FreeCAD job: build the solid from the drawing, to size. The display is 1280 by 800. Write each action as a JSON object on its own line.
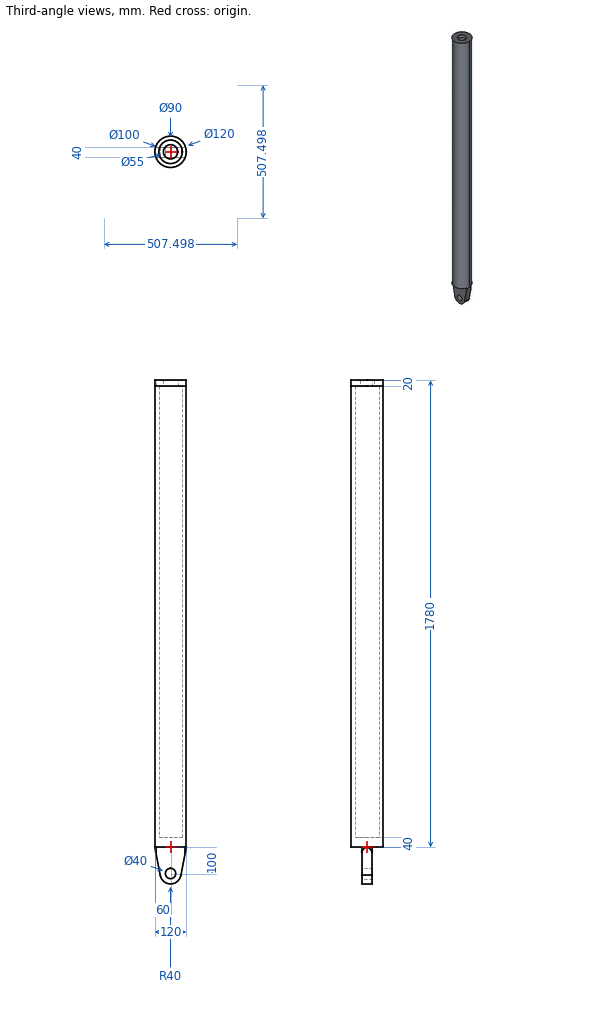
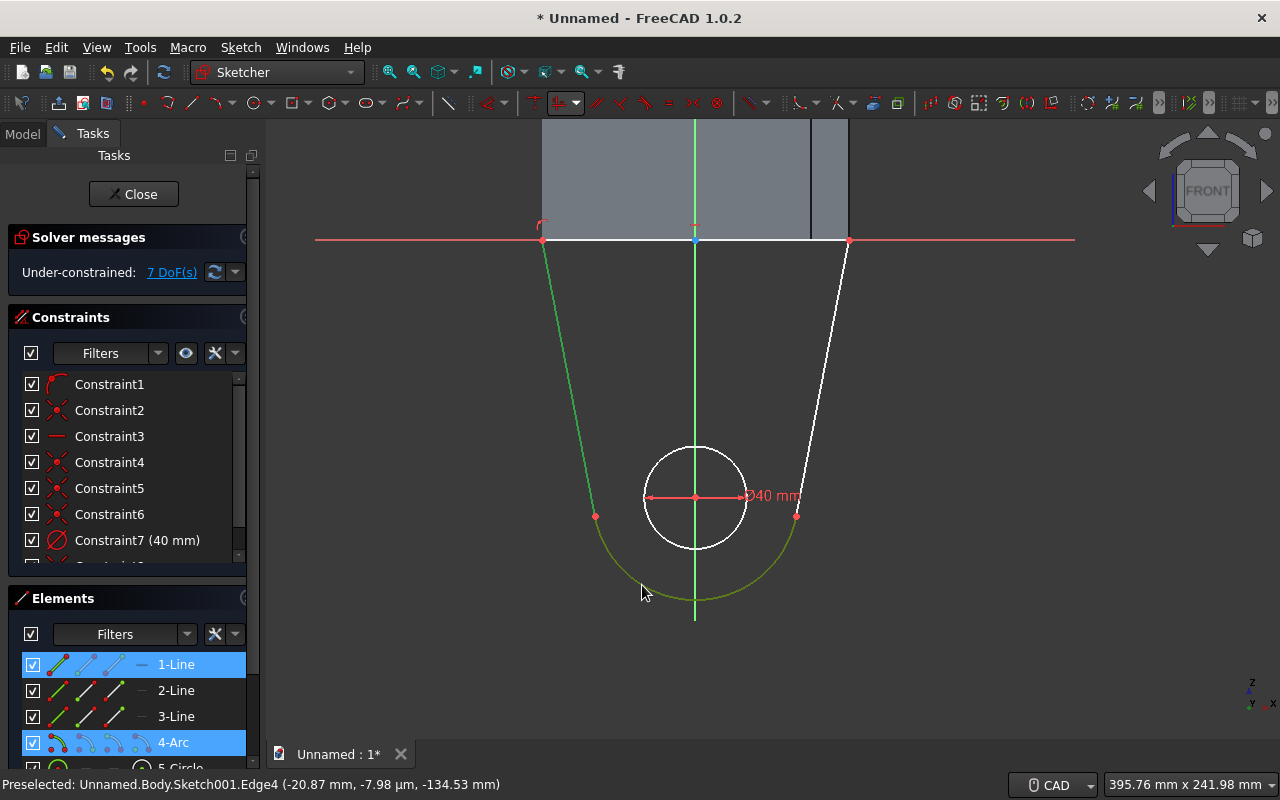
{"action": "left_click", "coordinate": [646, 104]}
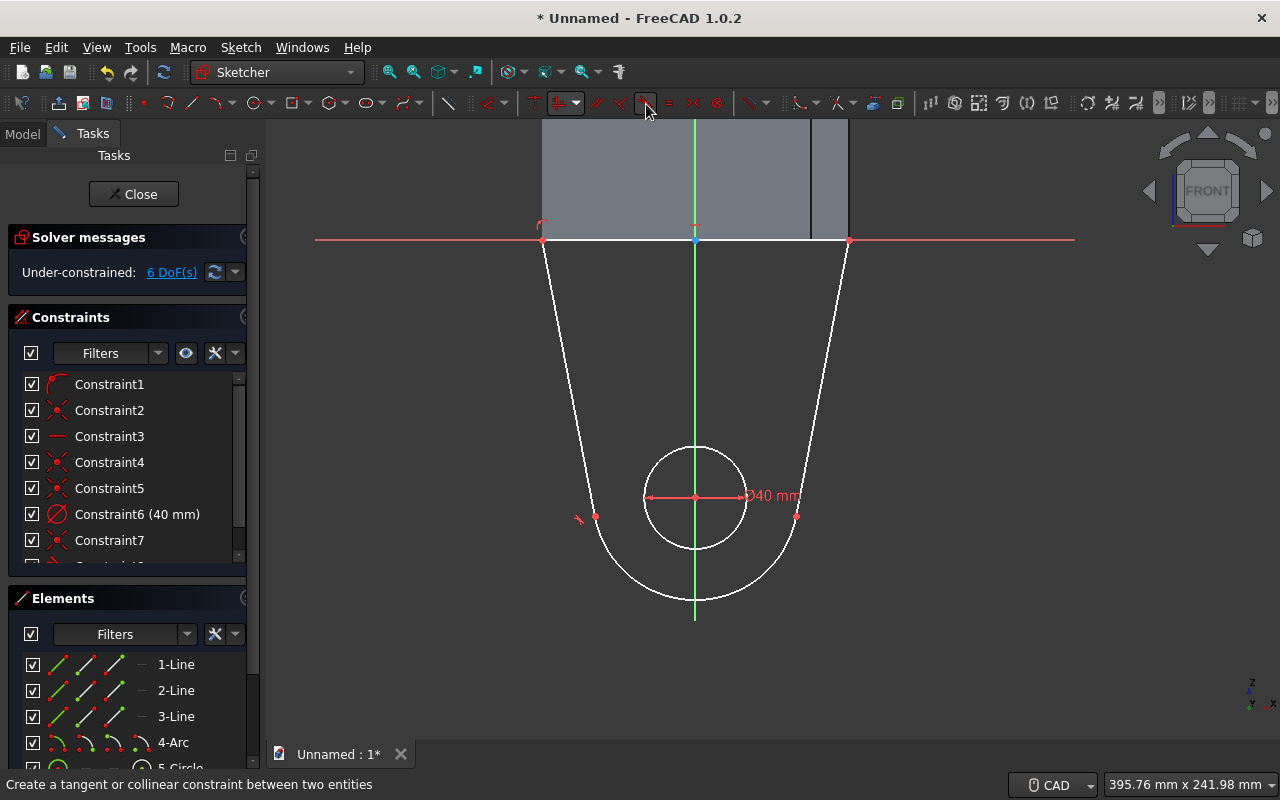
{"action": "left_click", "coordinate": [833, 323]}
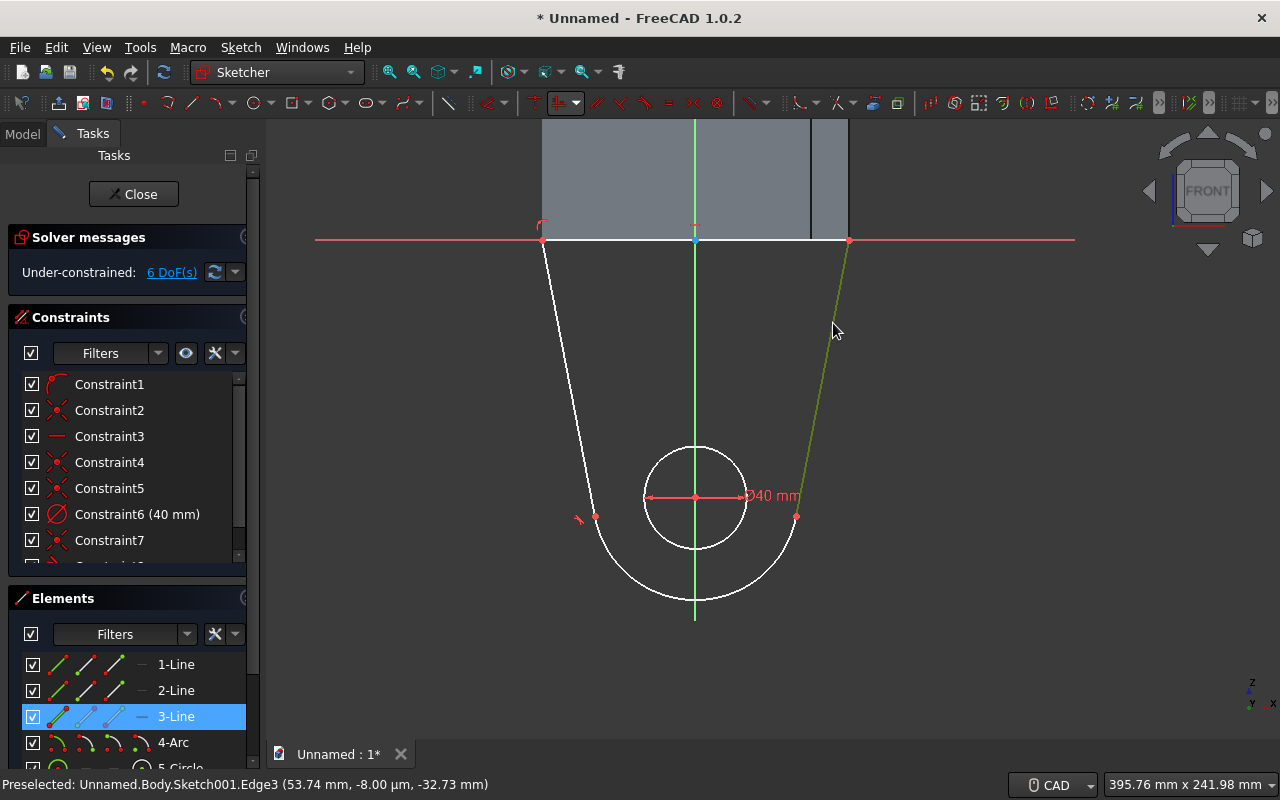
{"action": "left_click", "coordinate": [642, 585]}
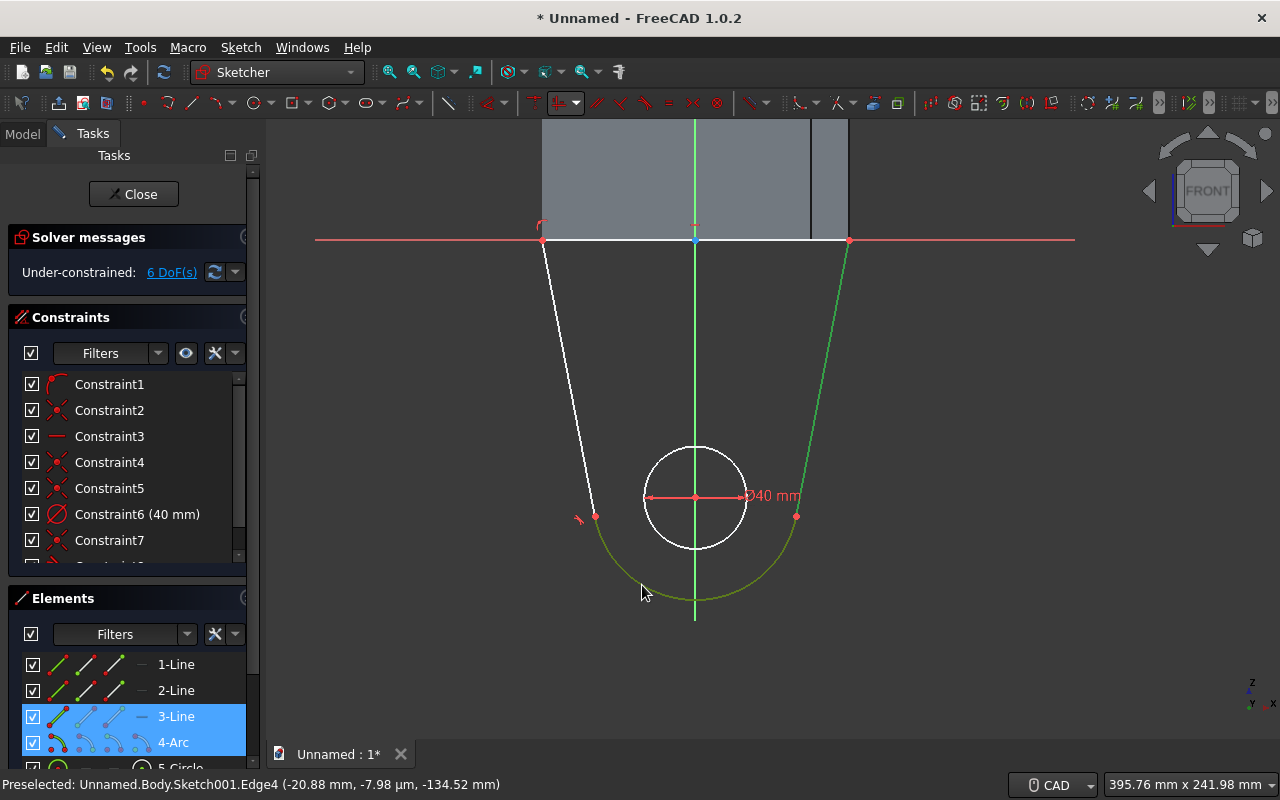
{"action": "key", "text": "t"}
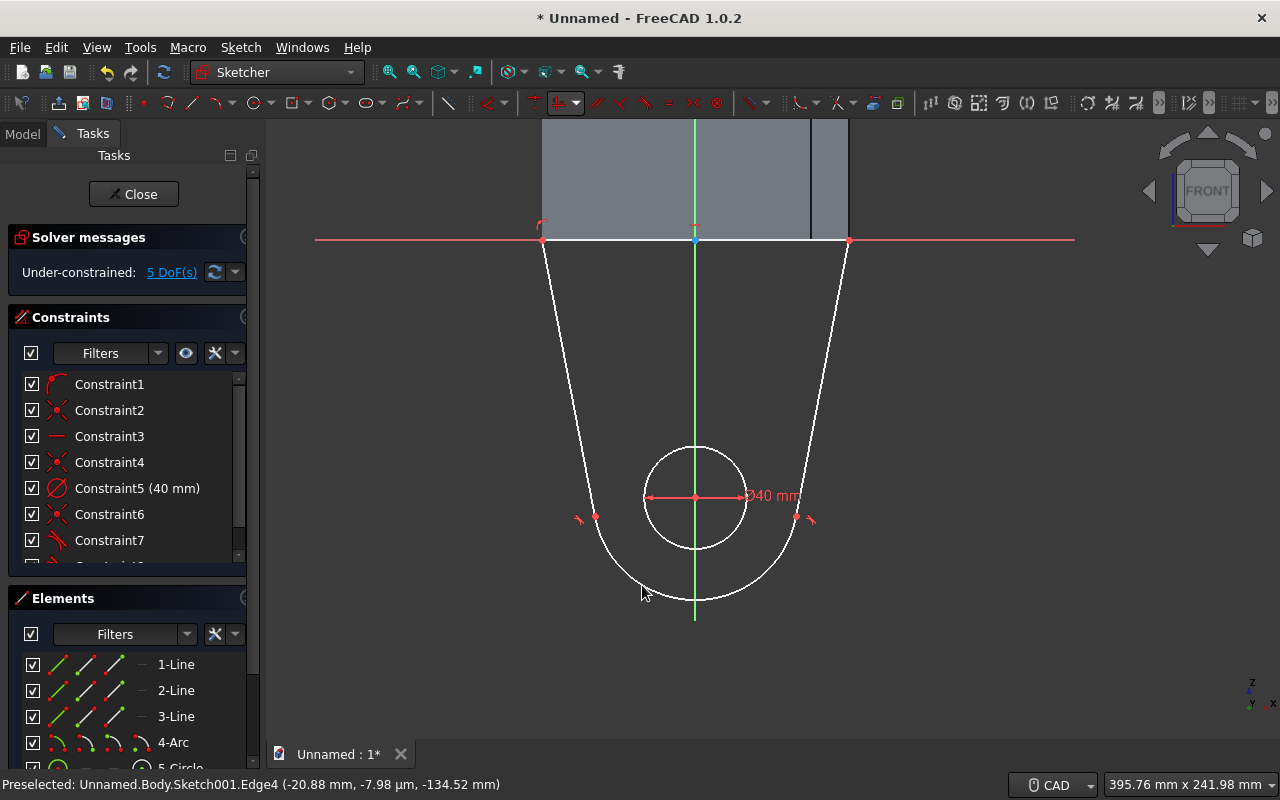
{"action": "left_click", "coordinate": [695, 498]}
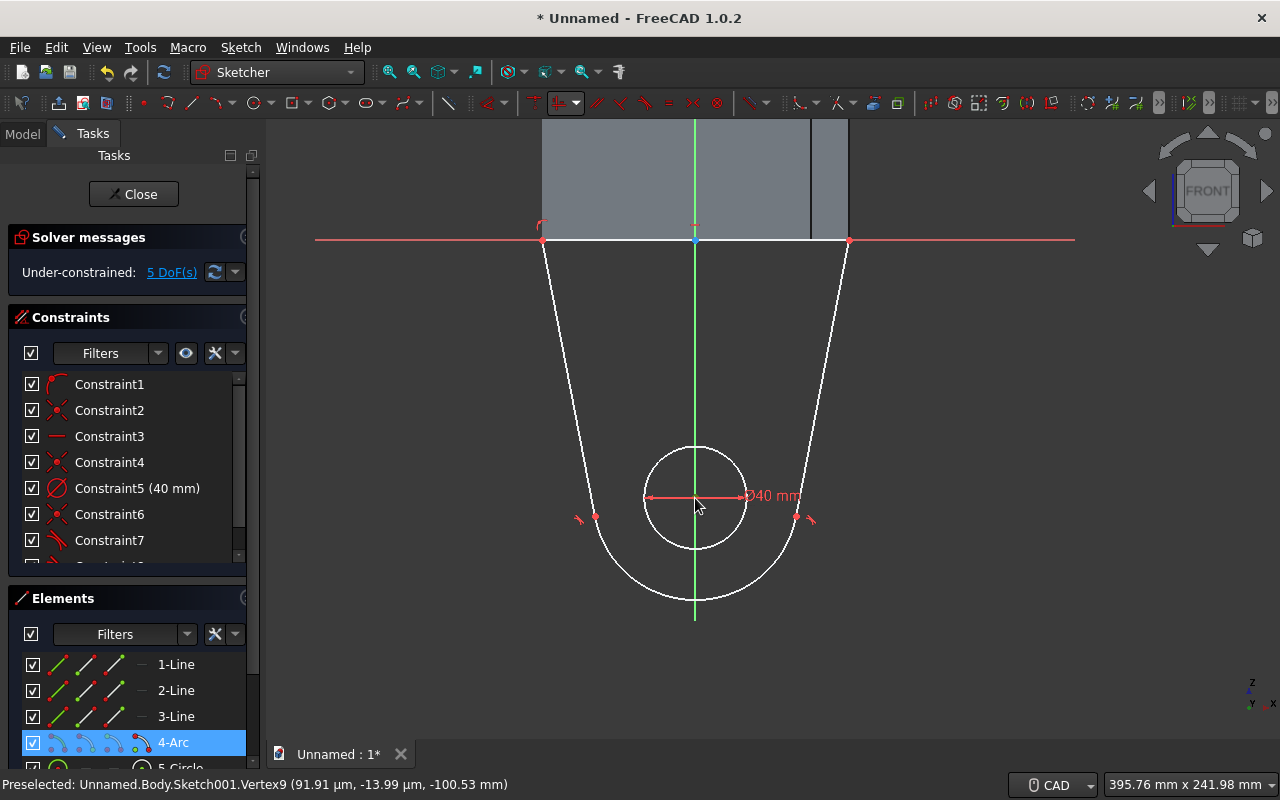
{"action": "left_click", "coordinate": [695, 510]}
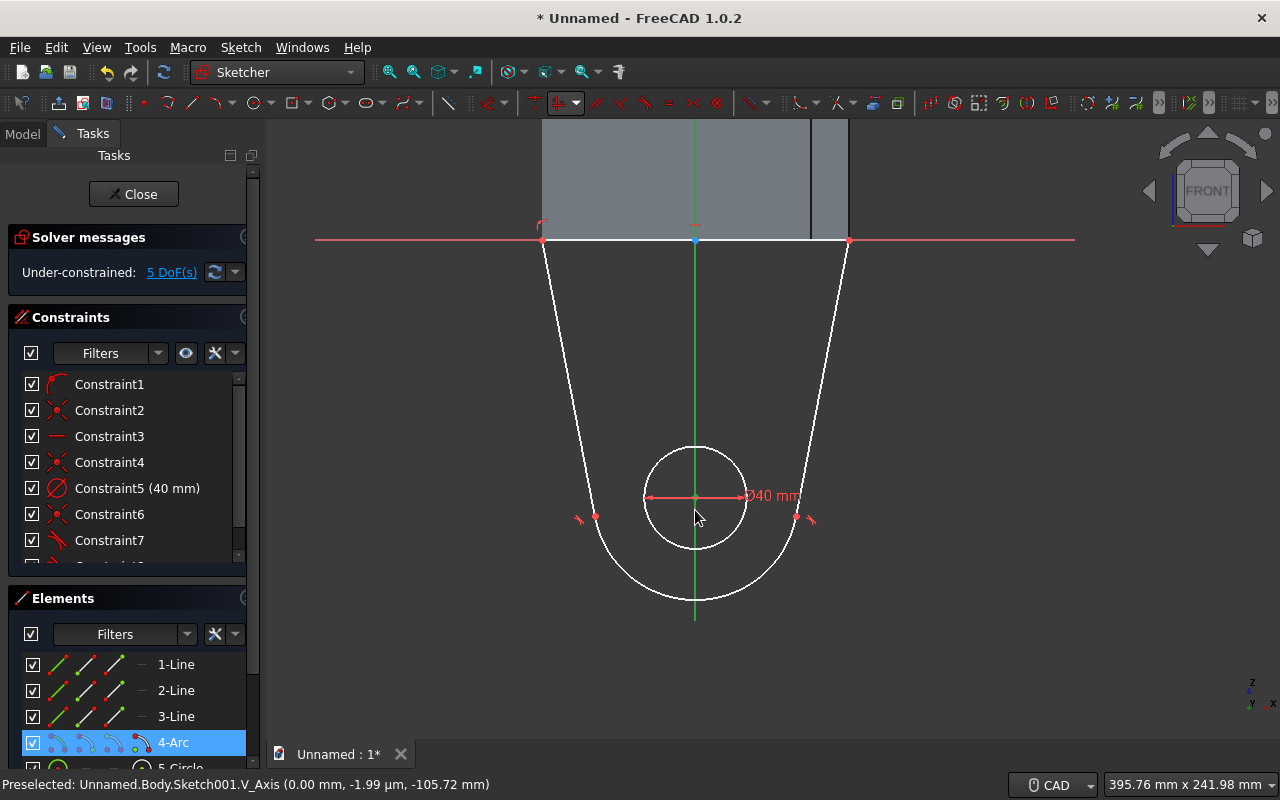
{"action": "left_click", "coordinate": [534, 104]}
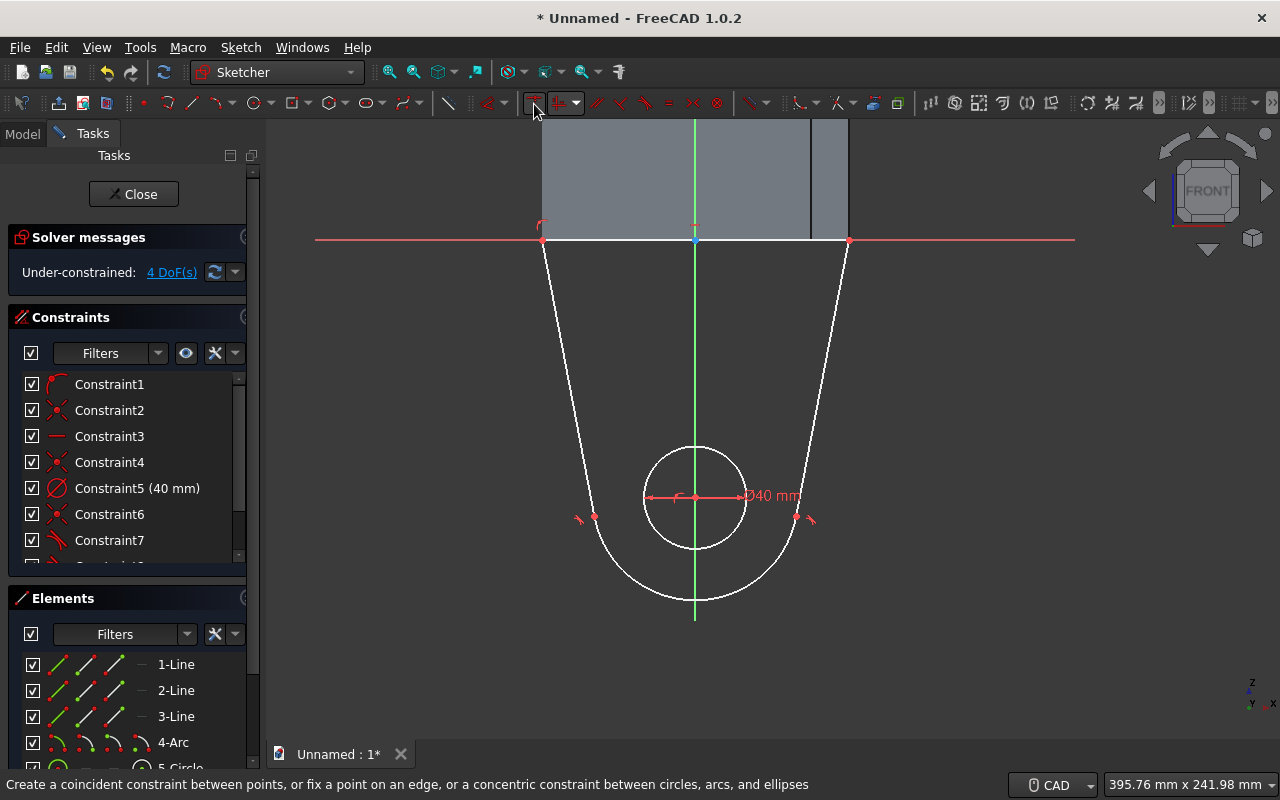
{"action": "left_click", "coordinate": [641, 585]}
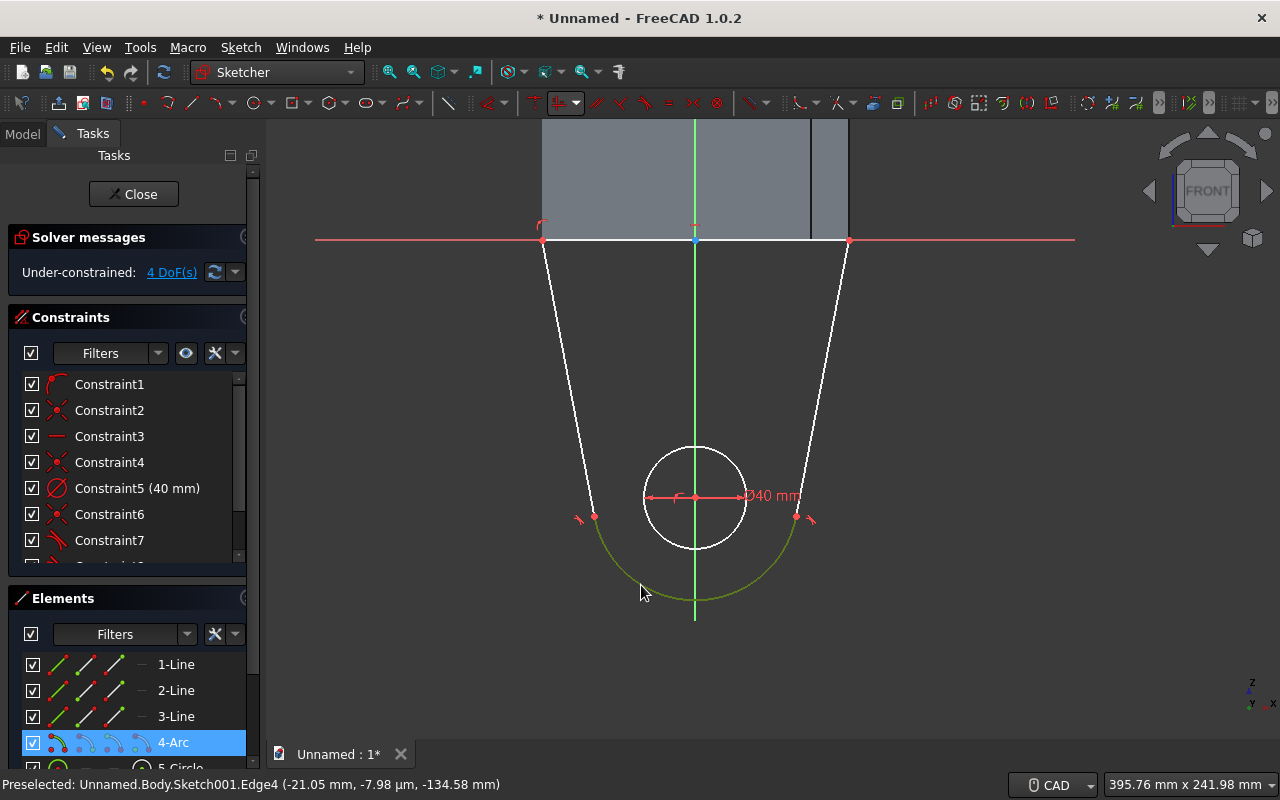
{"action": "left_click", "coordinate": [506, 104]}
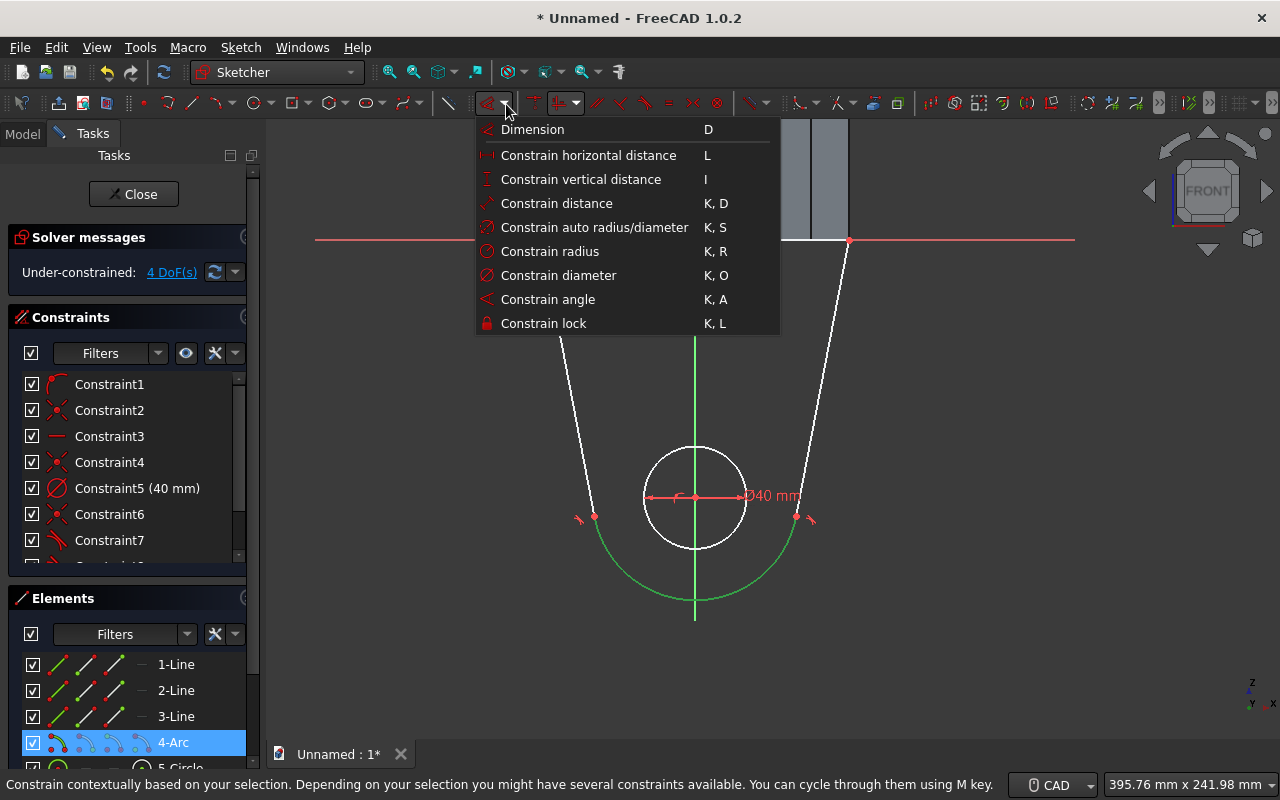
{"action": "left_click", "coordinate": [628, 251]}